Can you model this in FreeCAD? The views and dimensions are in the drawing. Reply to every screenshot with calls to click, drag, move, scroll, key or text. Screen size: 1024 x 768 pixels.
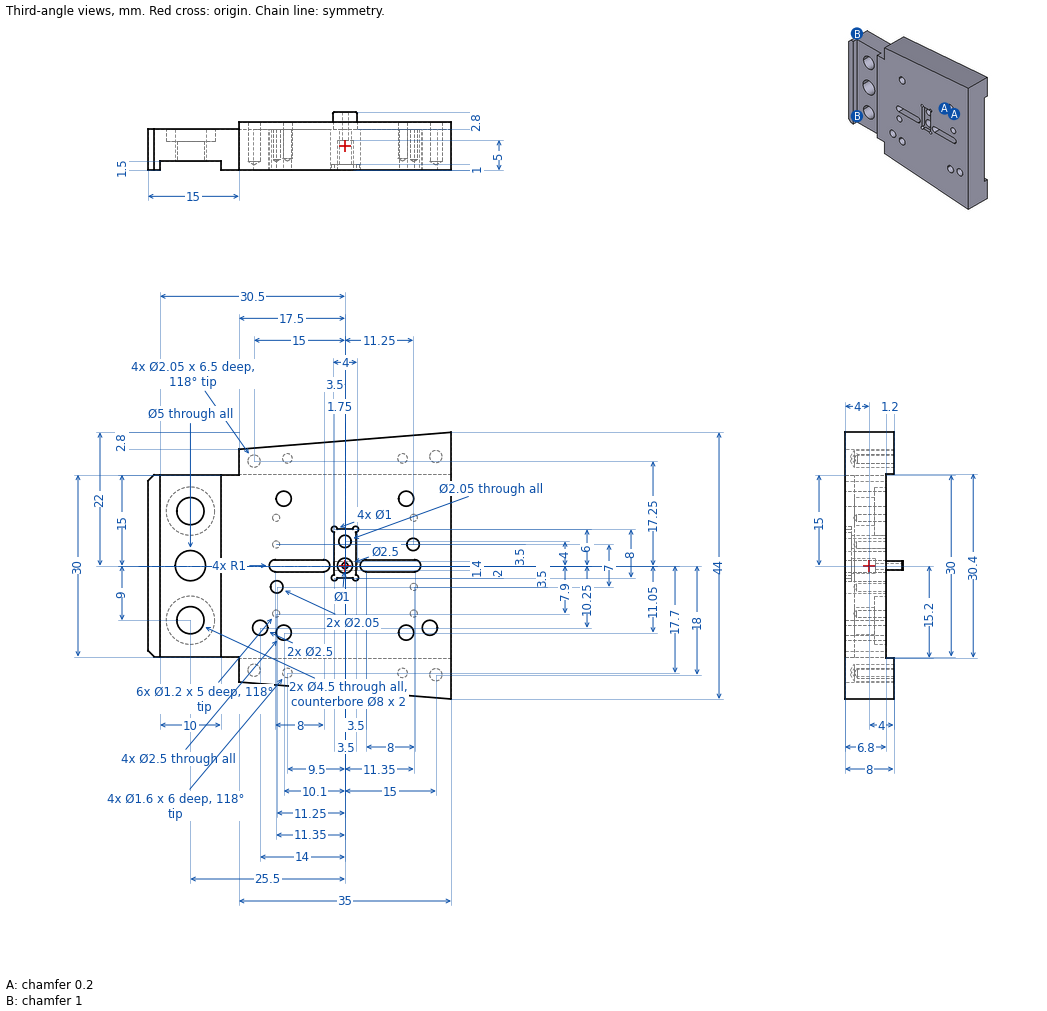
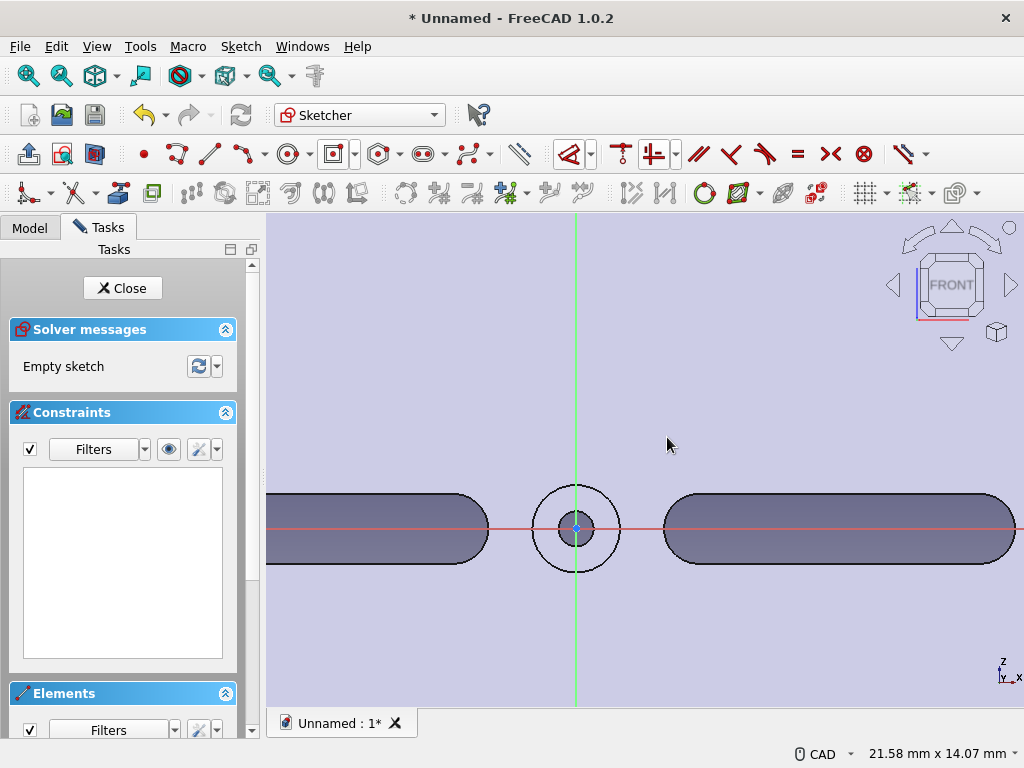
click(354, 154)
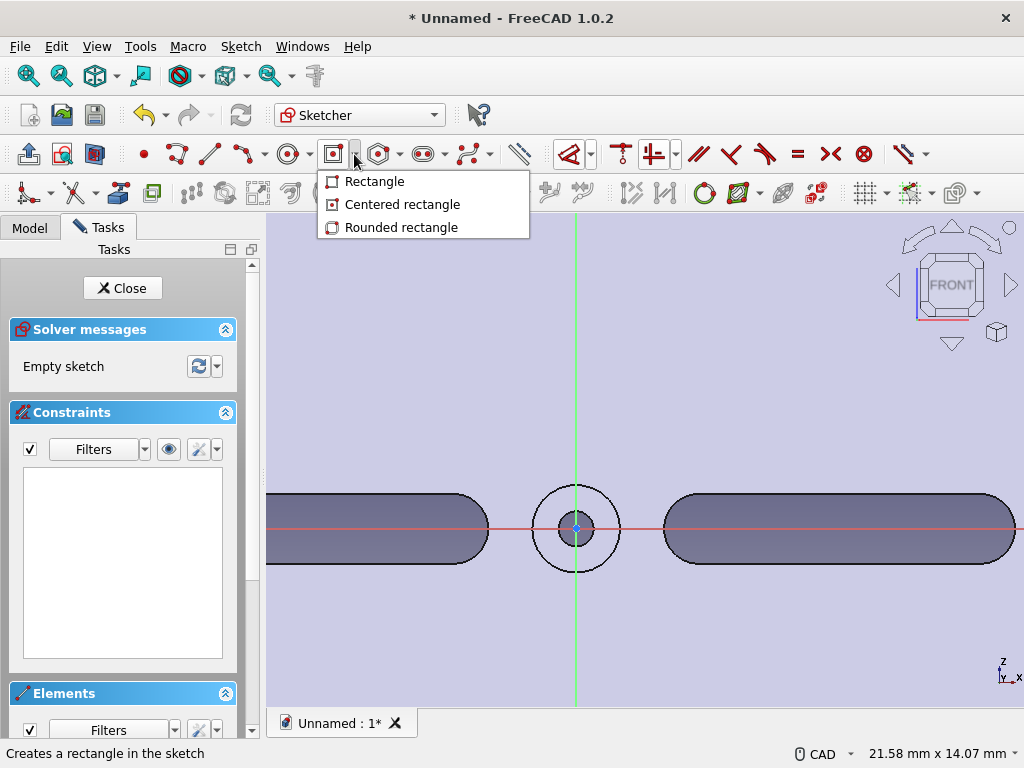
click(424, 182)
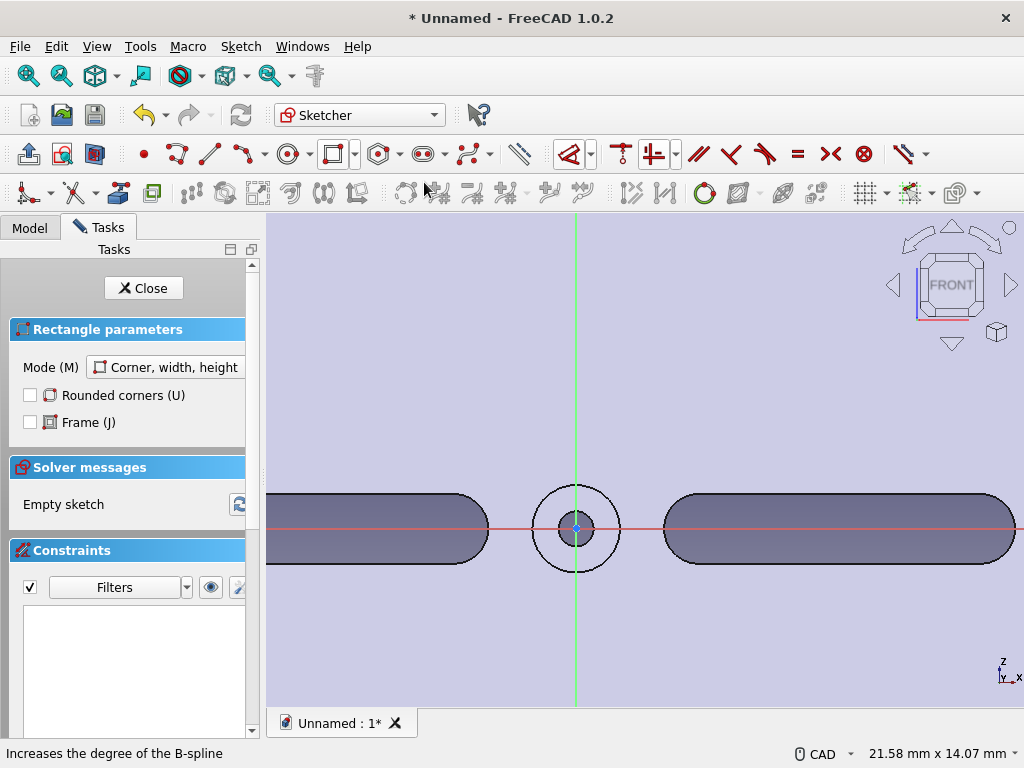
click(515, 318)
move(638, 599)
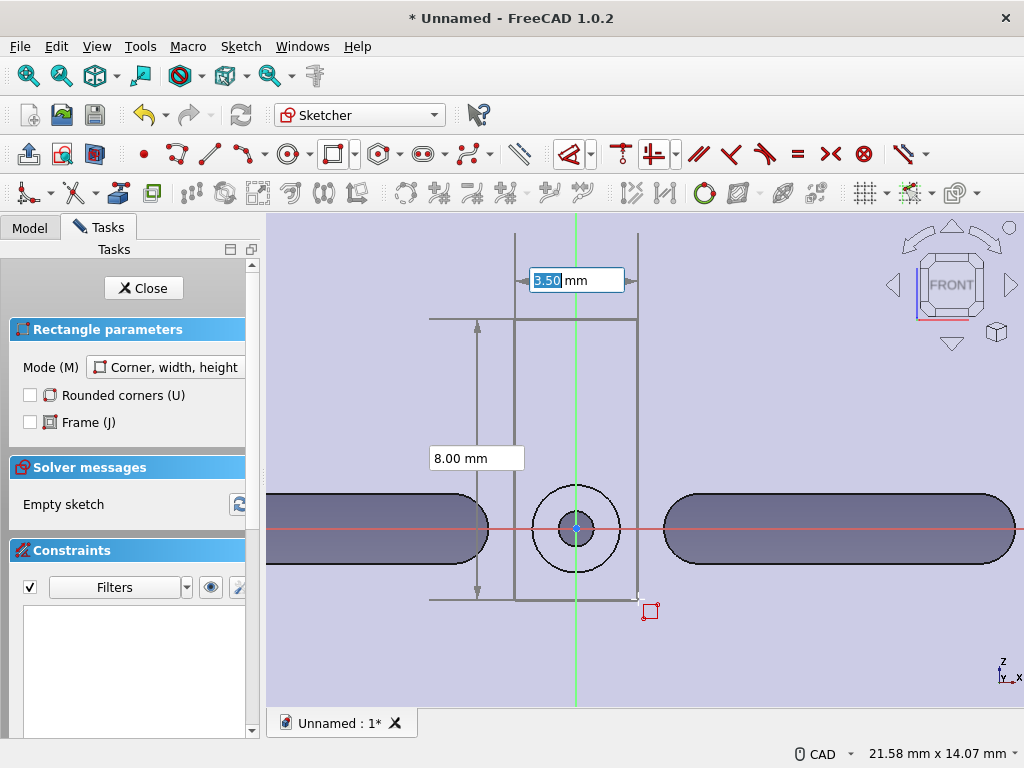
text(3.5)
key(Tab)
text(8)
key(Return)
key(Escape)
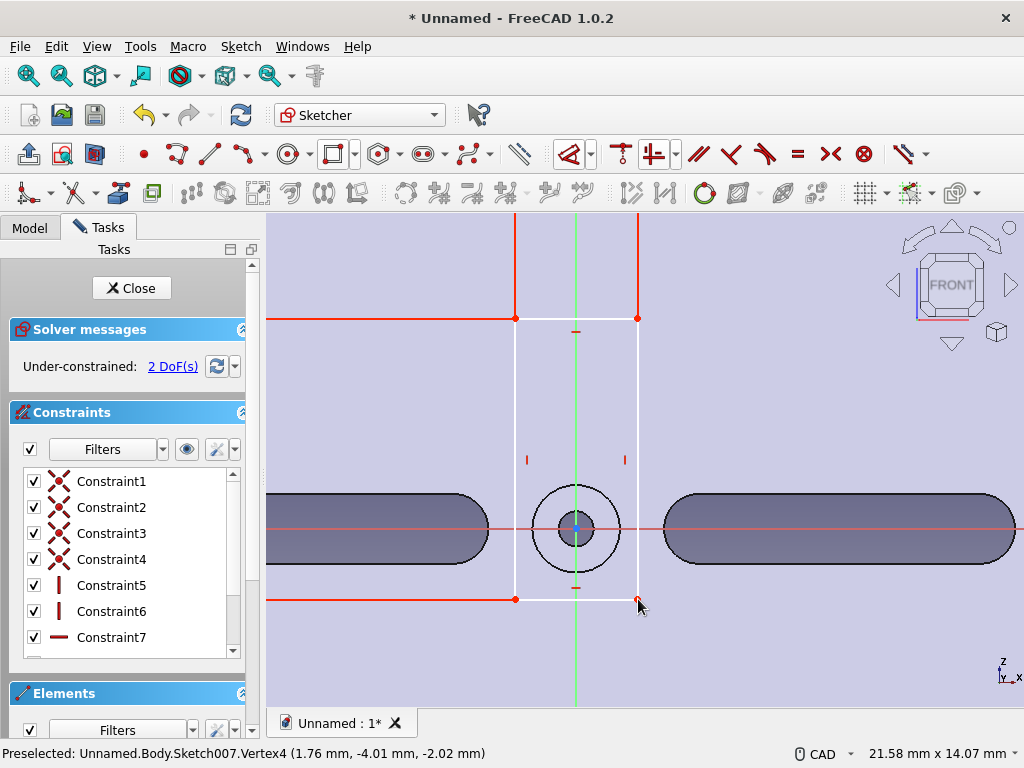
click(515, 319)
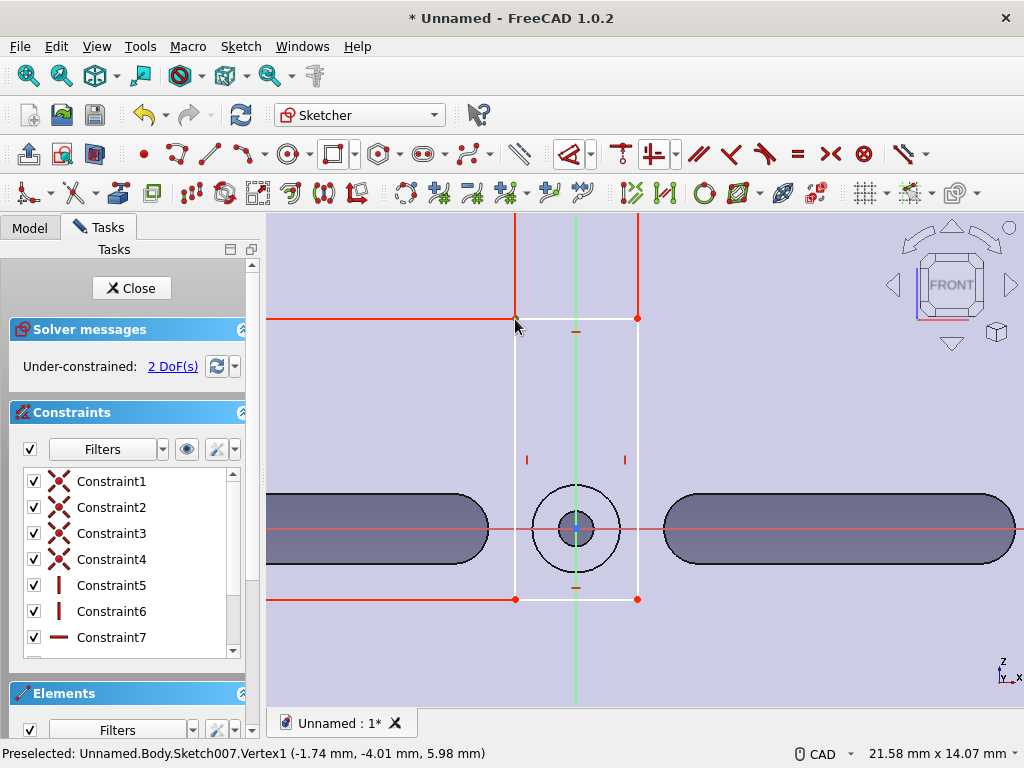
key(i)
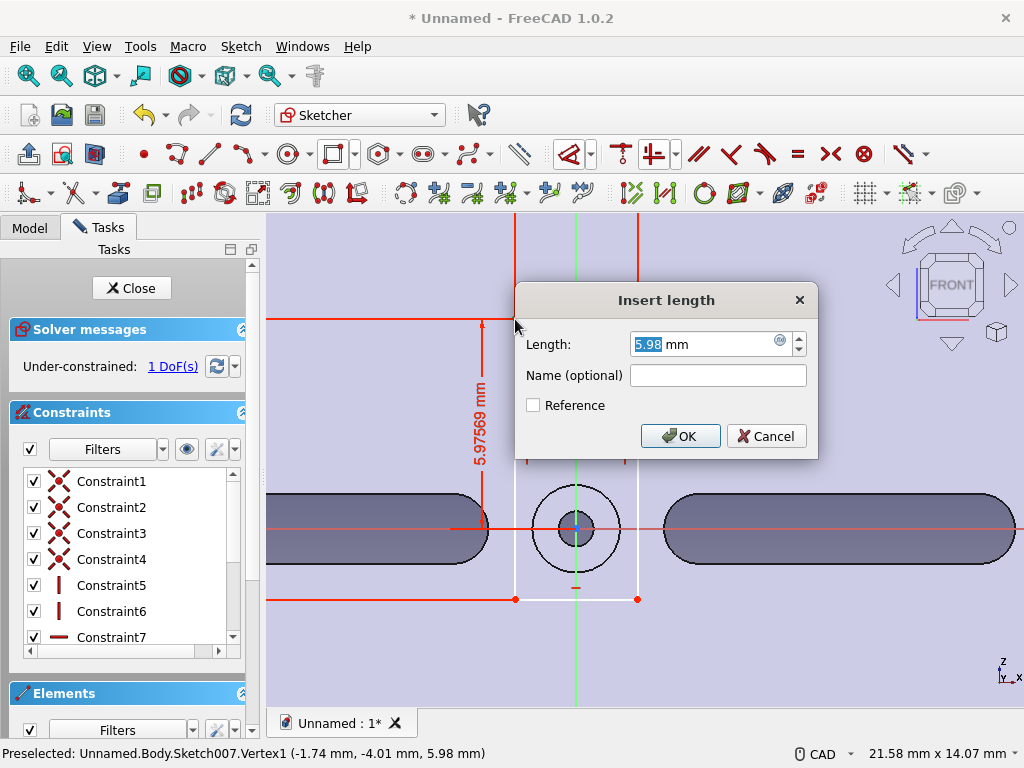
text(6)
key(Return)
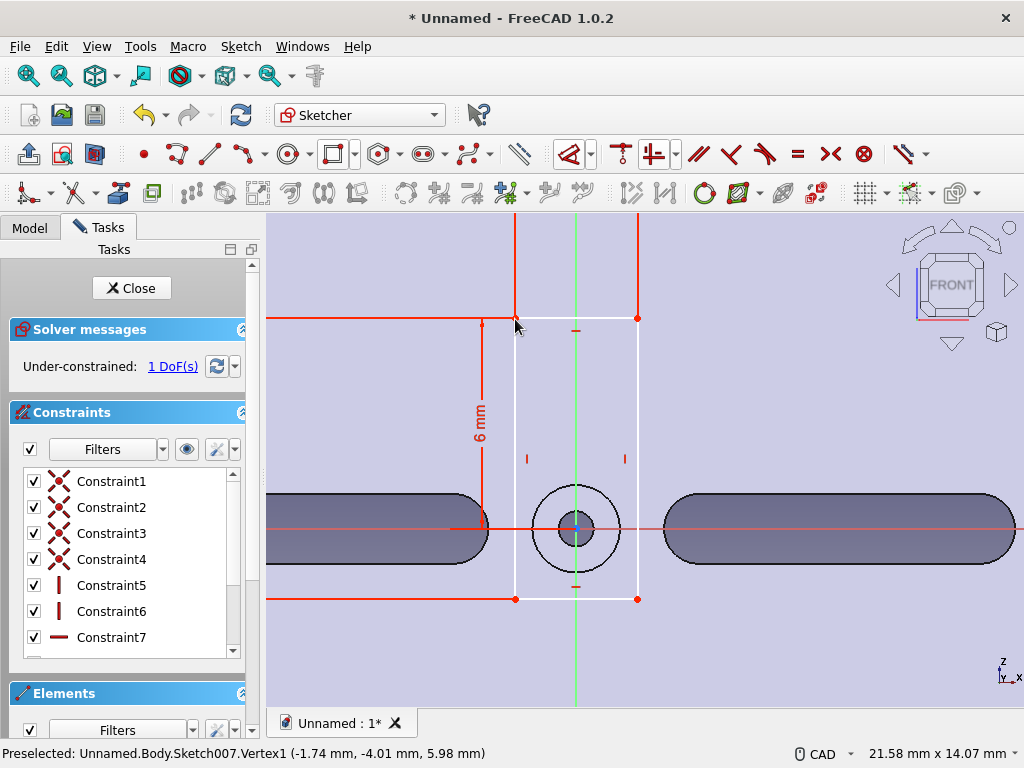
click(515, 318)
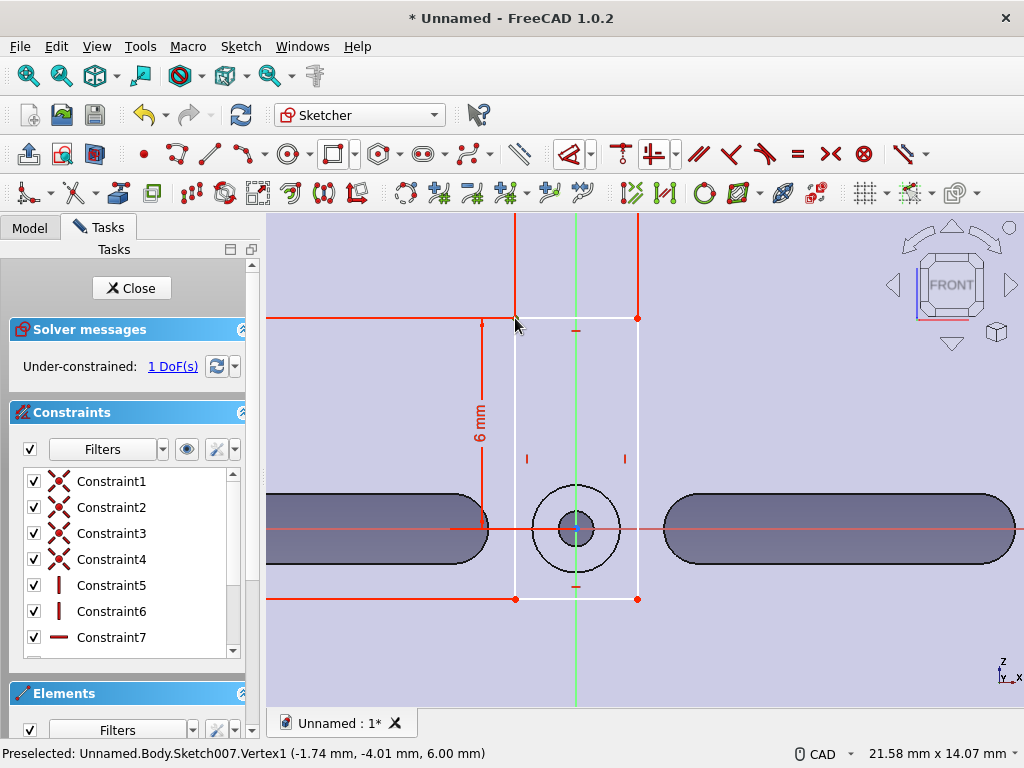
click(590, 154)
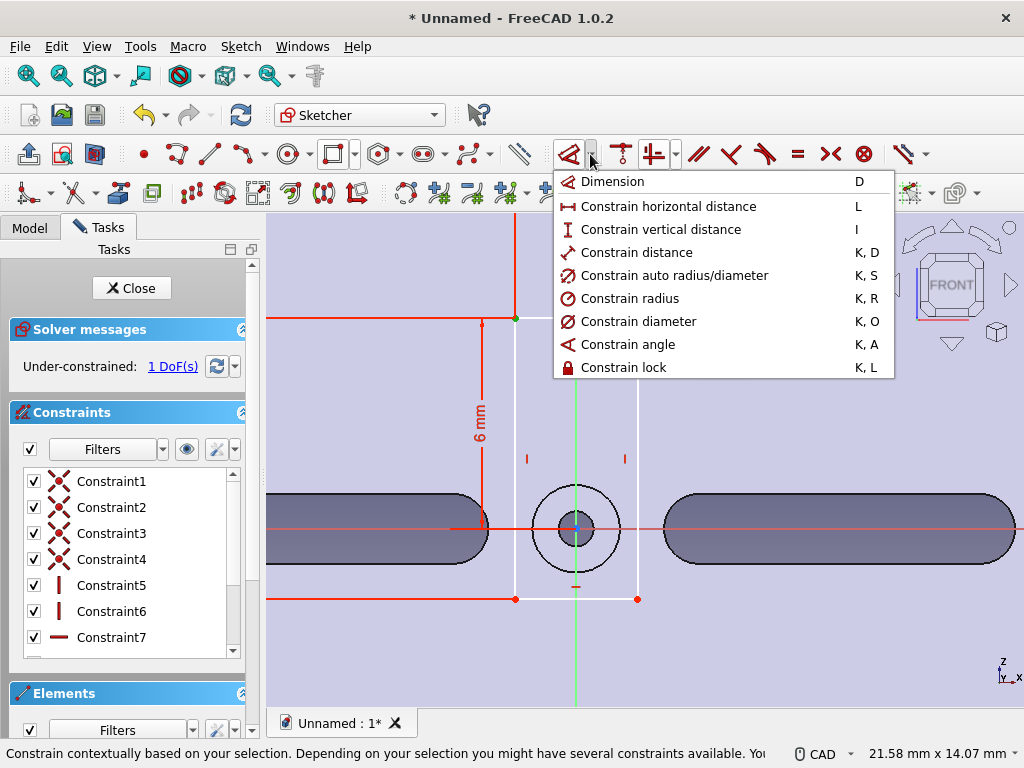
click(724, 206)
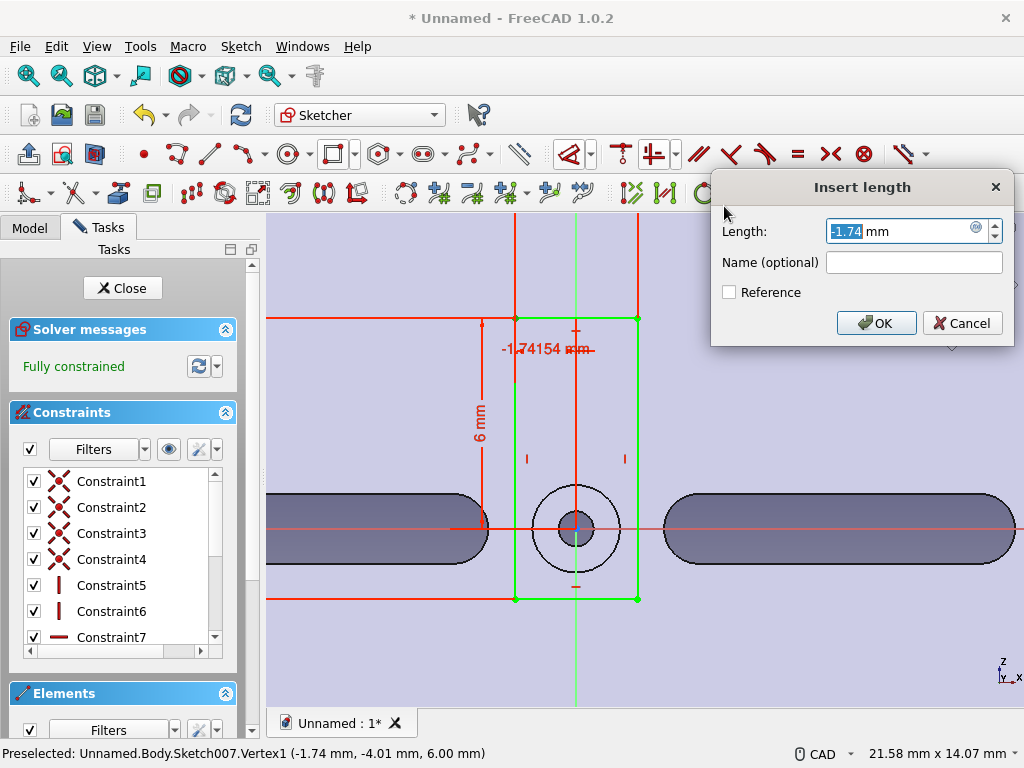
text(-1.75)
key(Return)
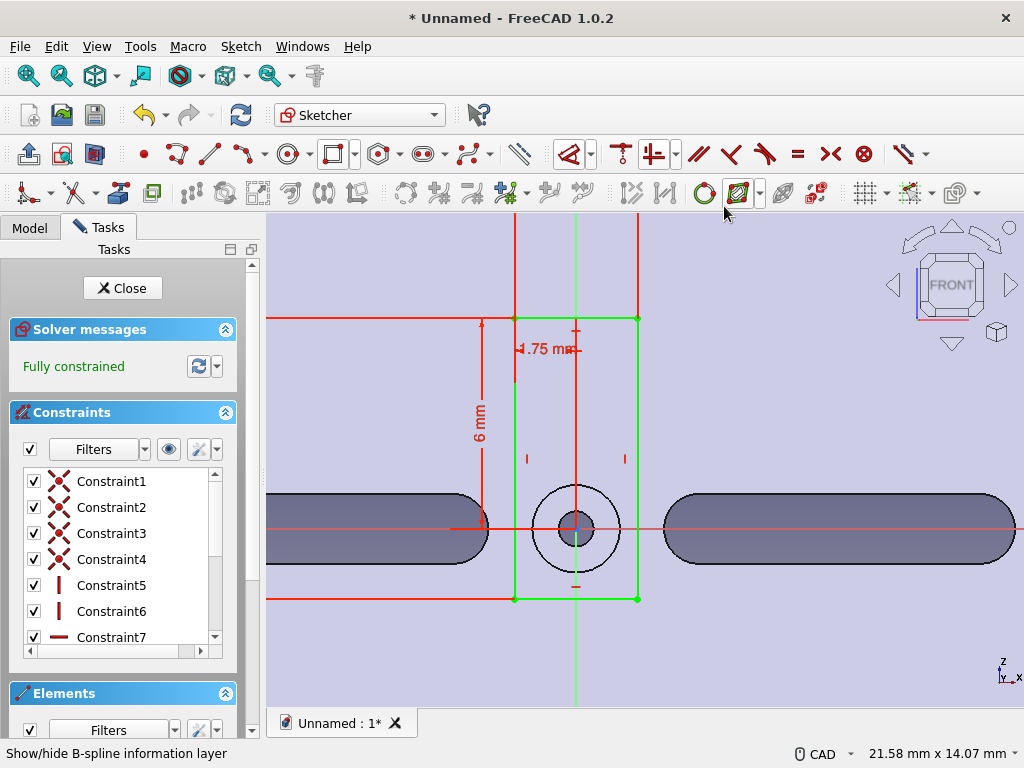
click(123, 288)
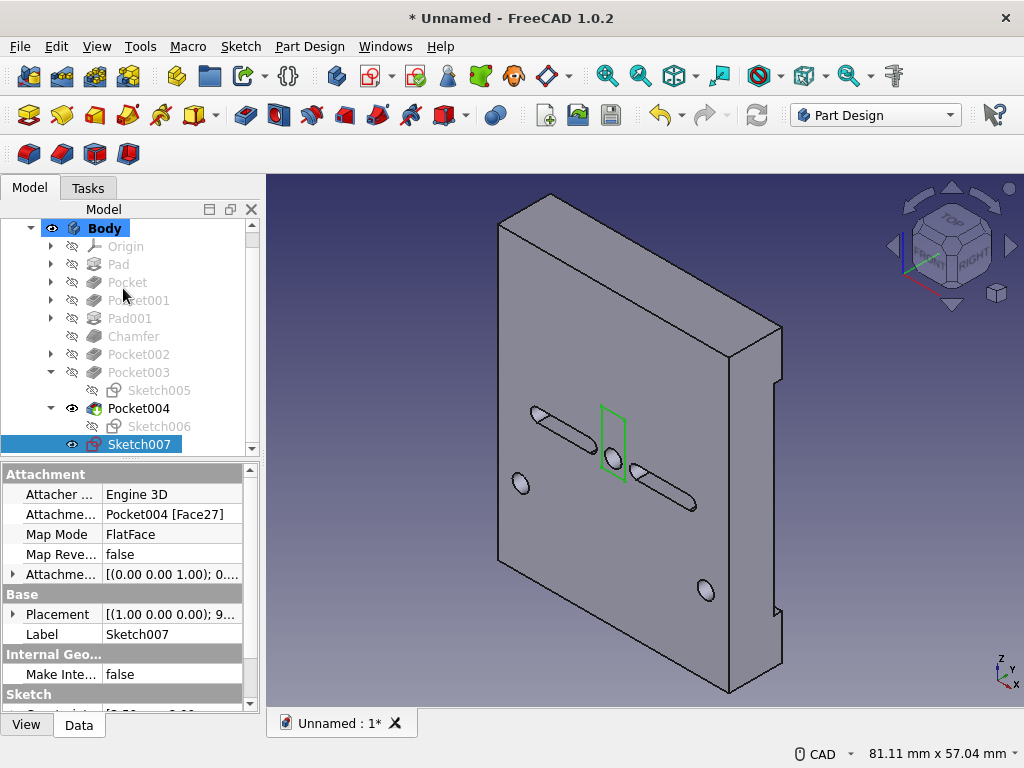
click(246, 116)